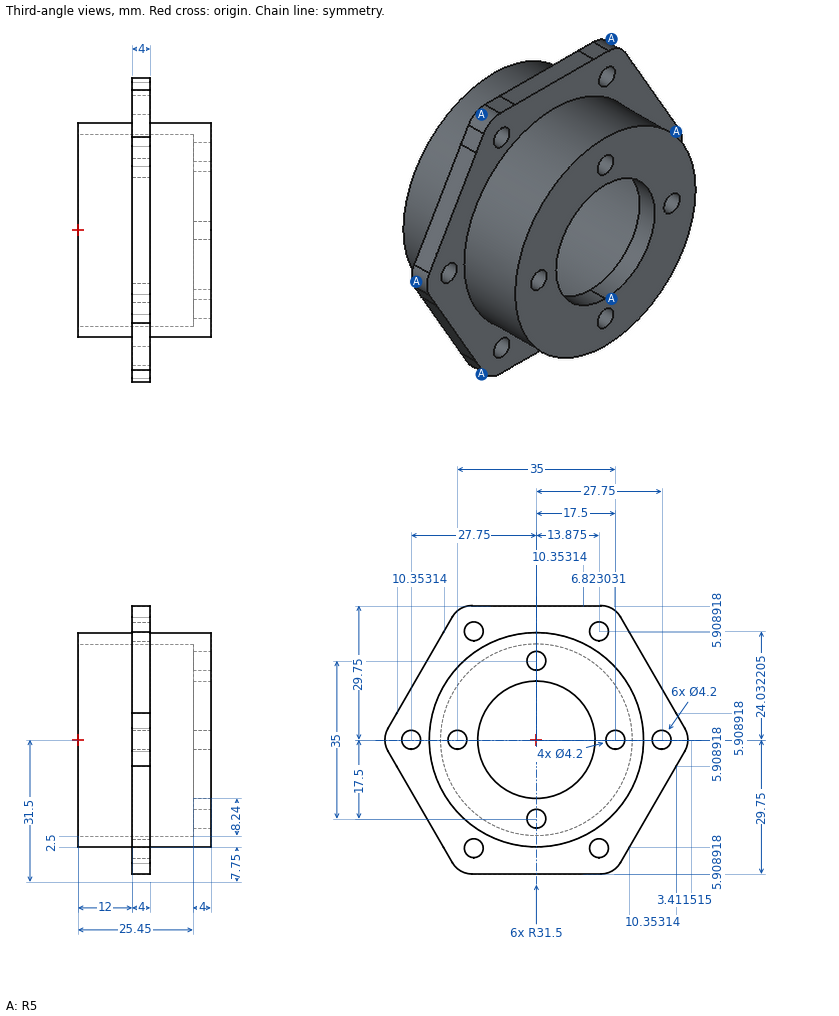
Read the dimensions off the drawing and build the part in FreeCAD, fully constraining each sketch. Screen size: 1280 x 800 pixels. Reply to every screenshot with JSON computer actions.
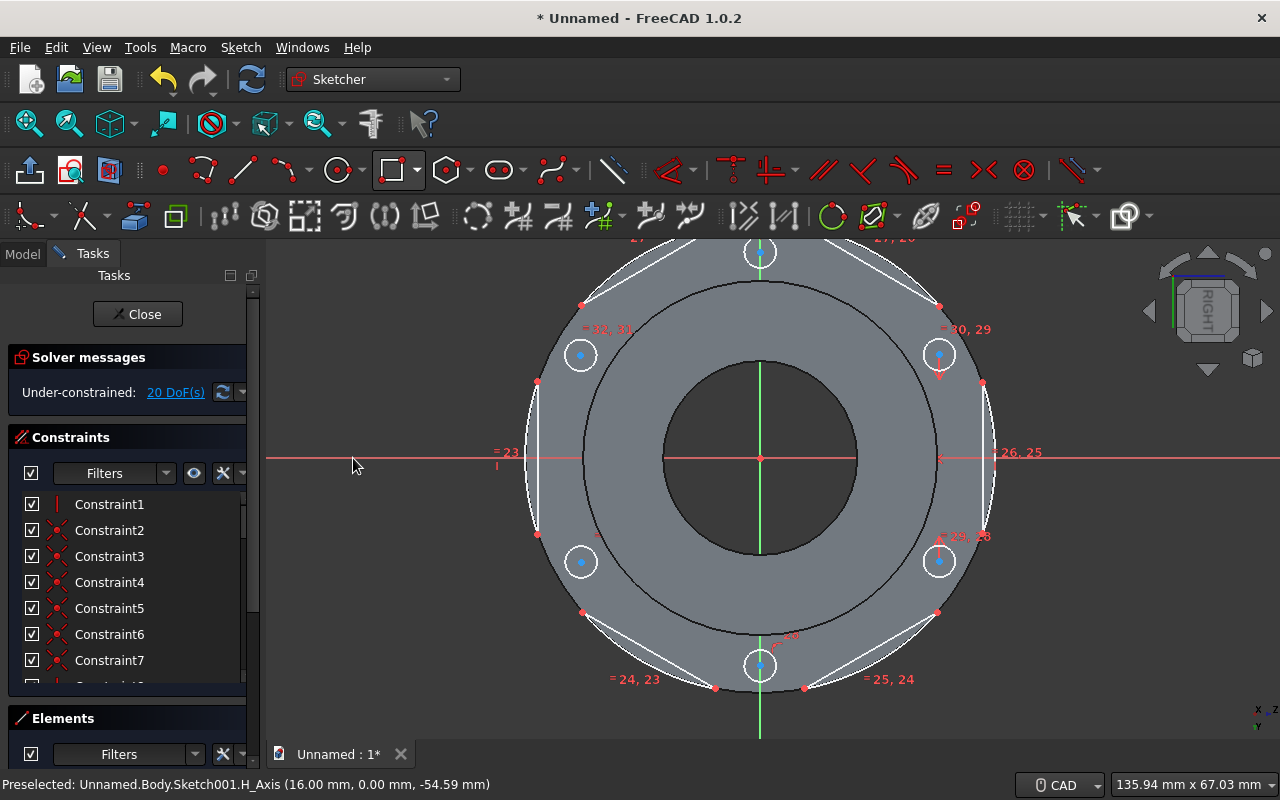
{"action": "left_click", "coordinate": [939, 355]}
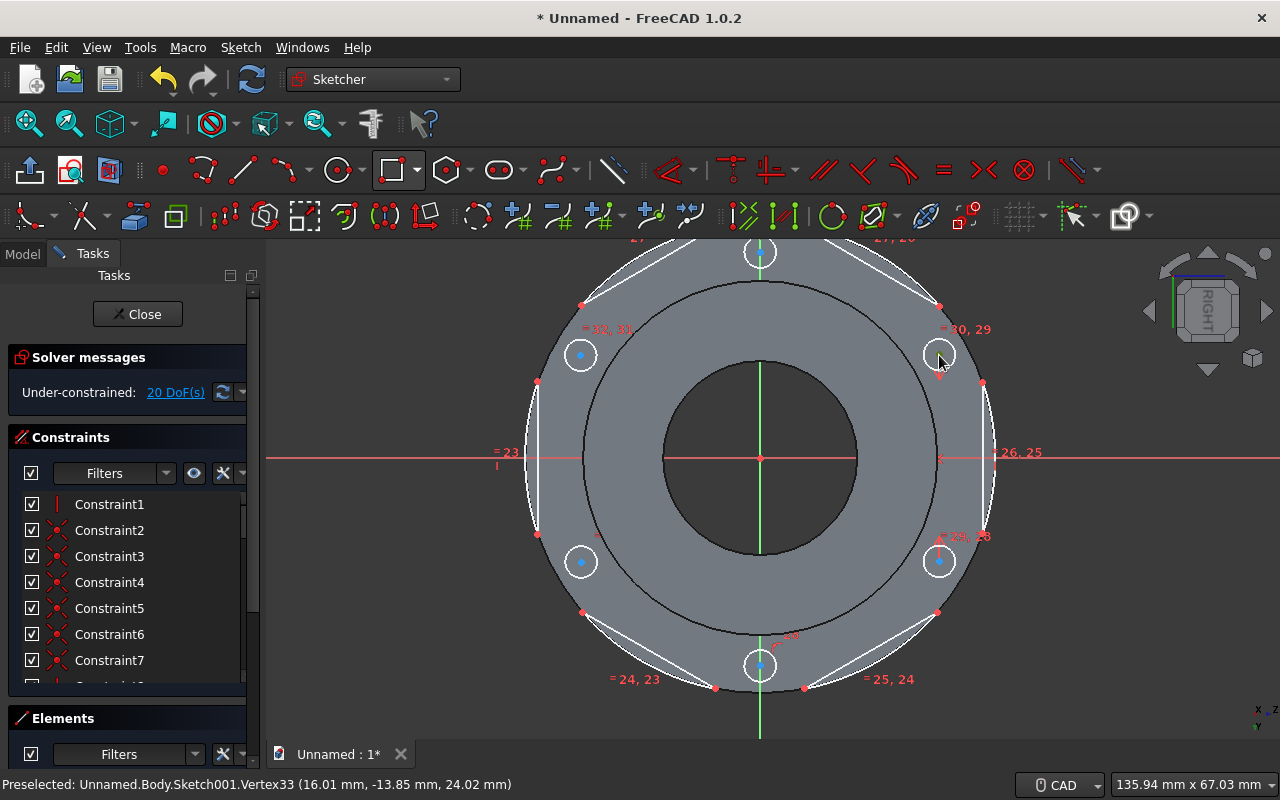
{"action": "left_click", "coordinate": [581, 355]}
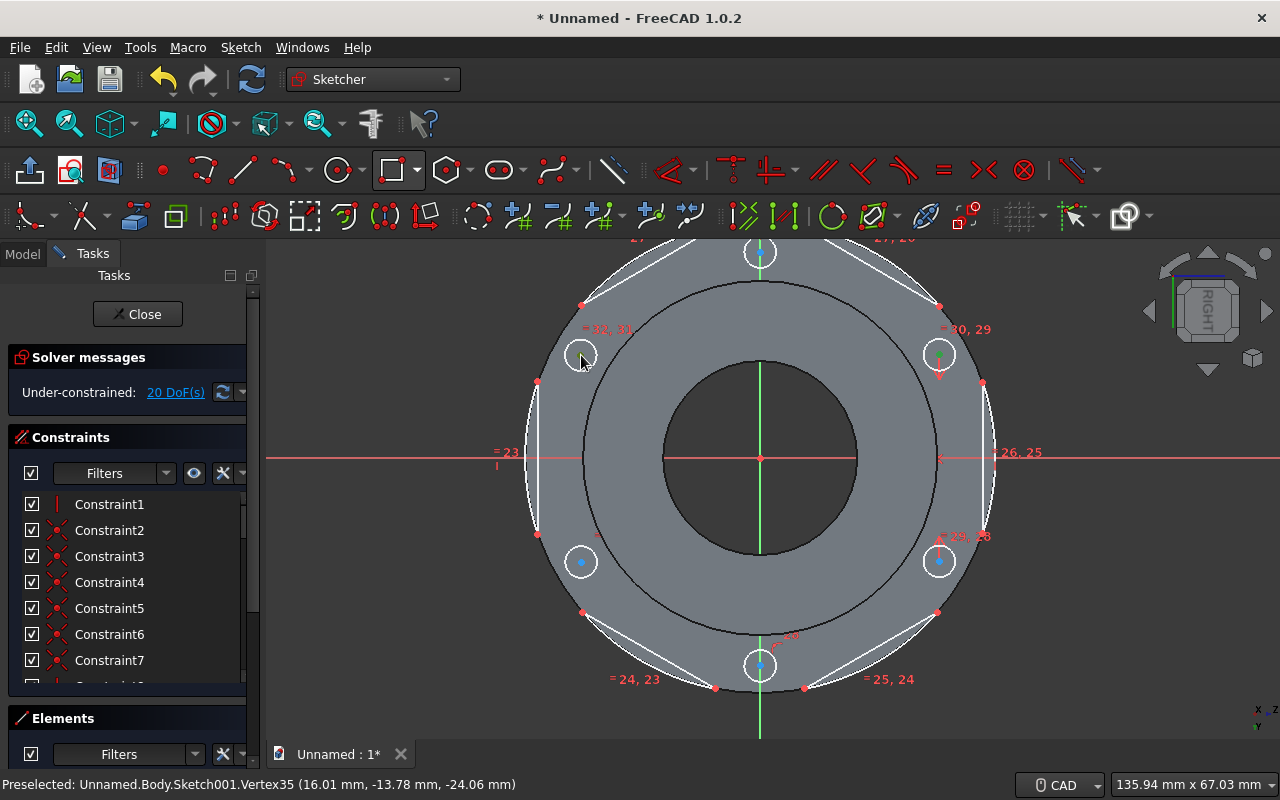
{"action": "left_click", "coordinate": [760, 616]}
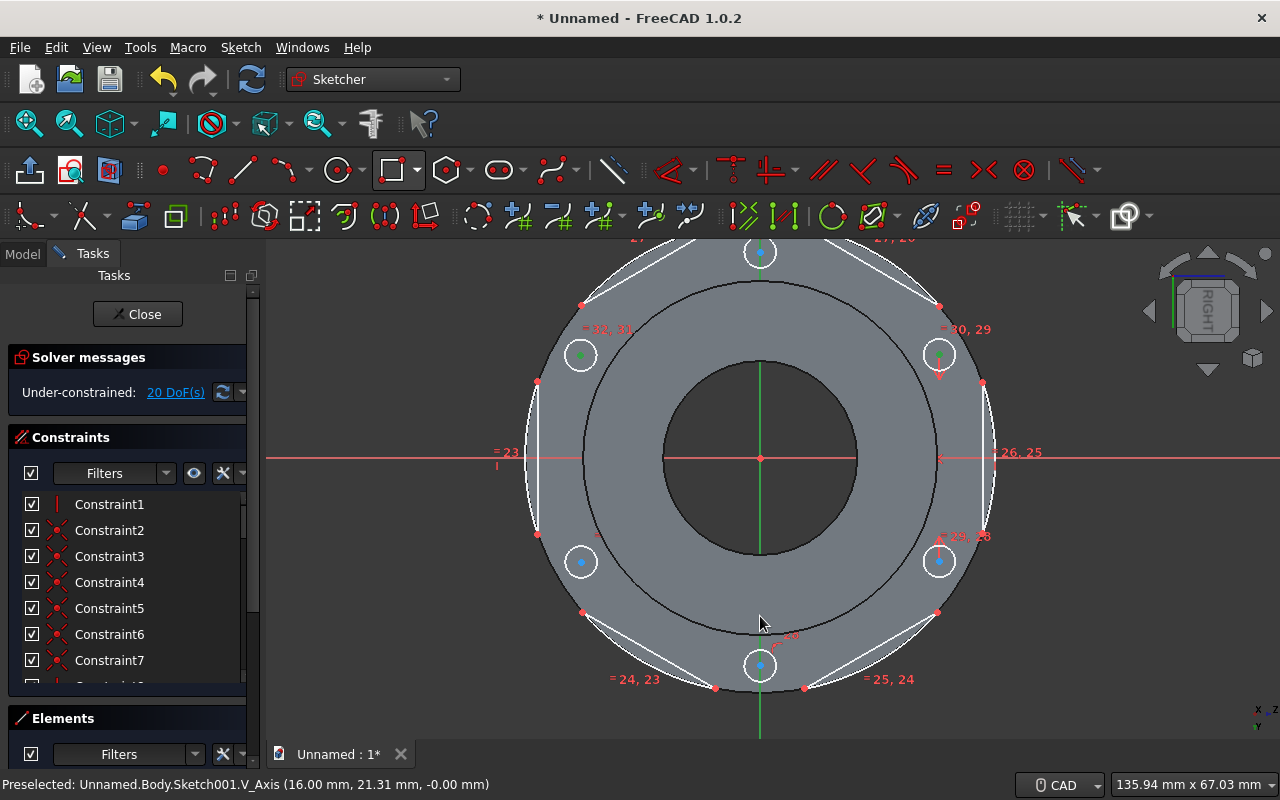
{"action": "key", "text": "s"}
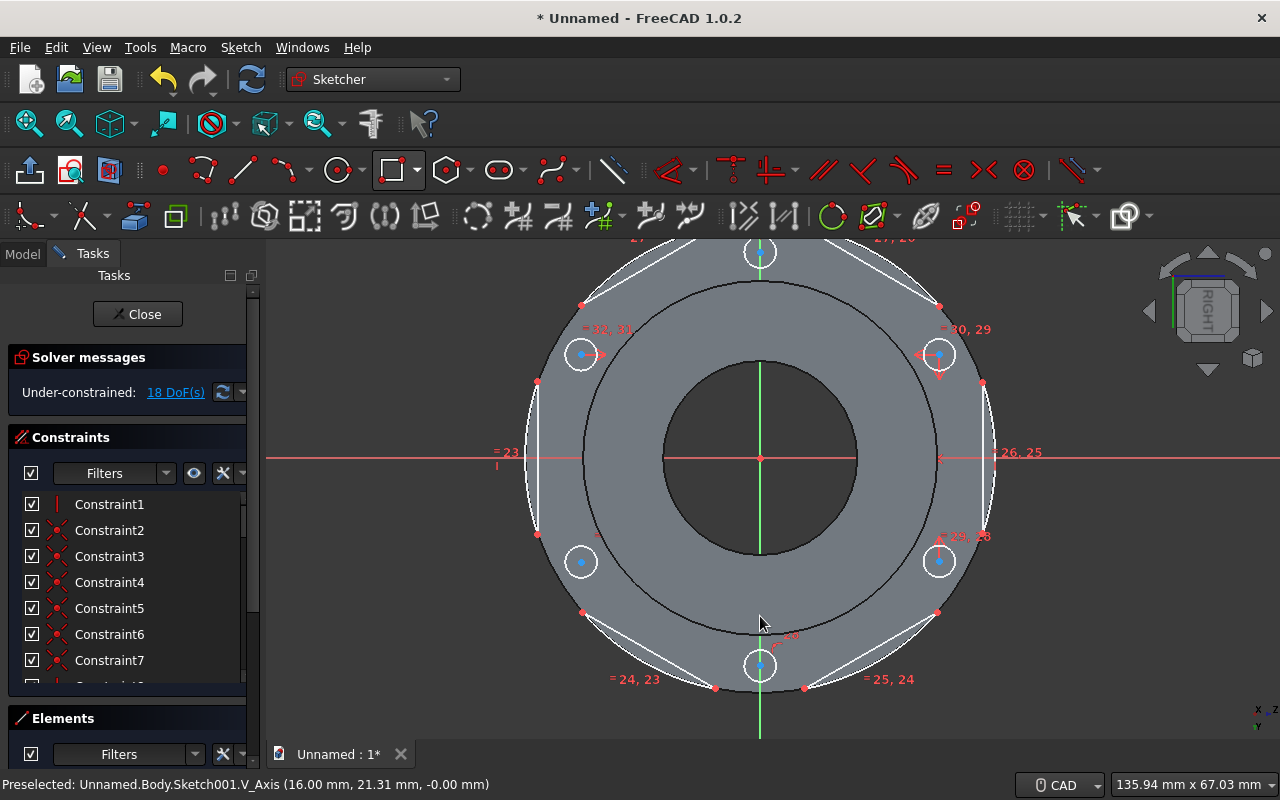
{"action": "left_click", "coordinate": [939, 561]}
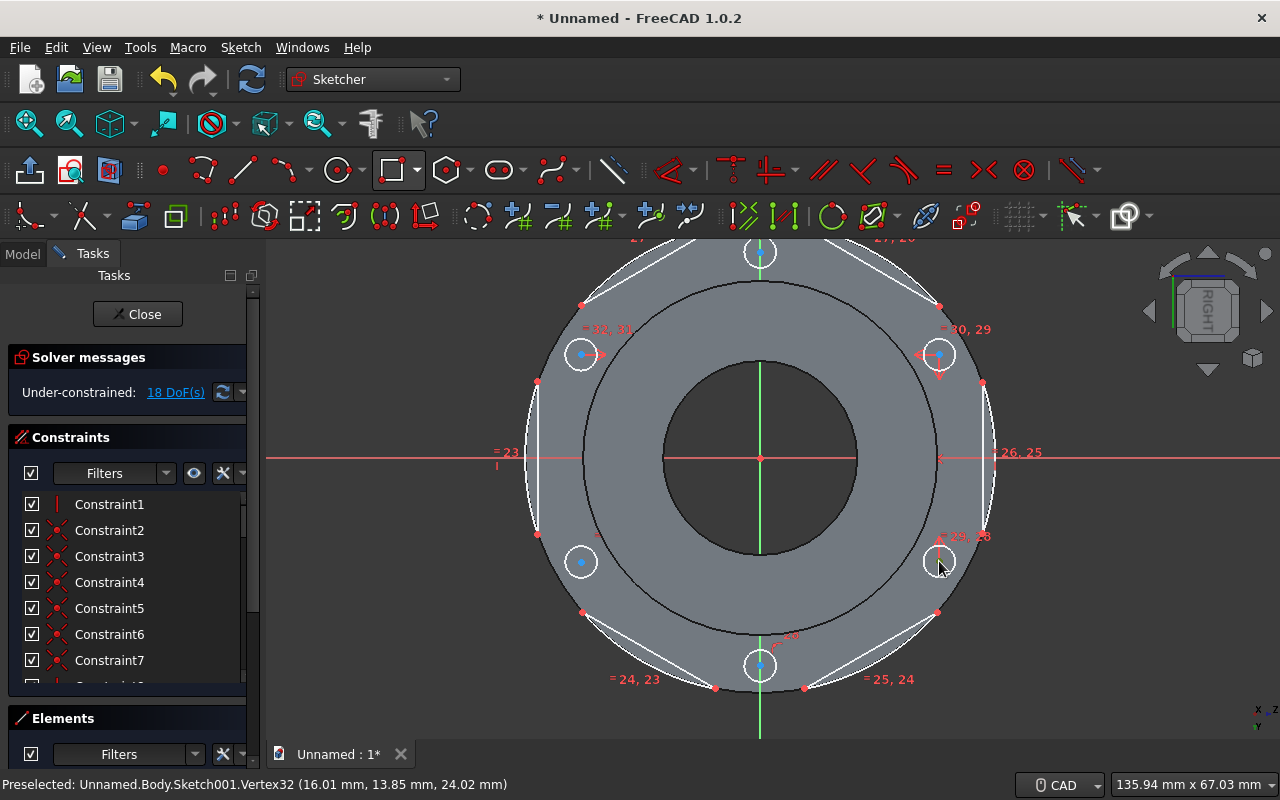
{"action": "left_click", "coordinate": [581, 562]}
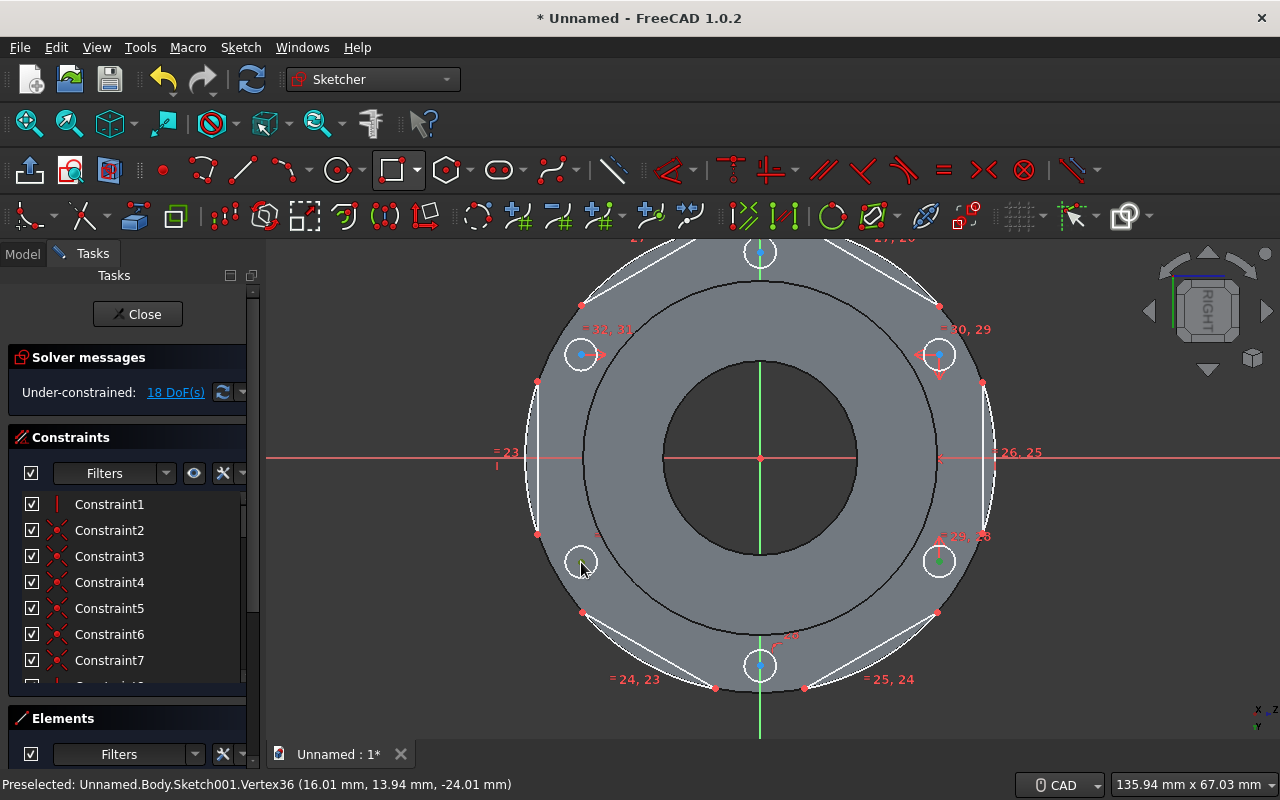
{"action": "left_click", "coordinate": [760, 616]}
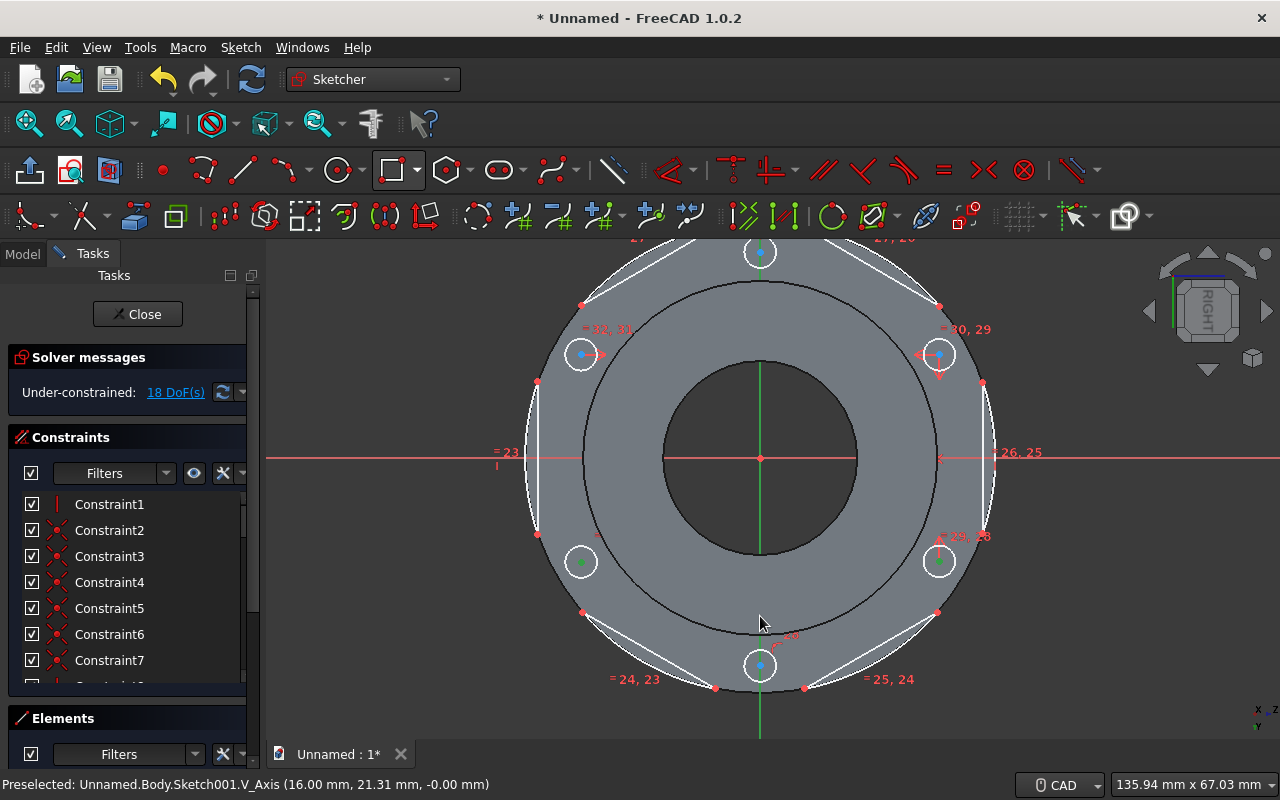
{"action": "left_click", "coordinate": [984, 170]}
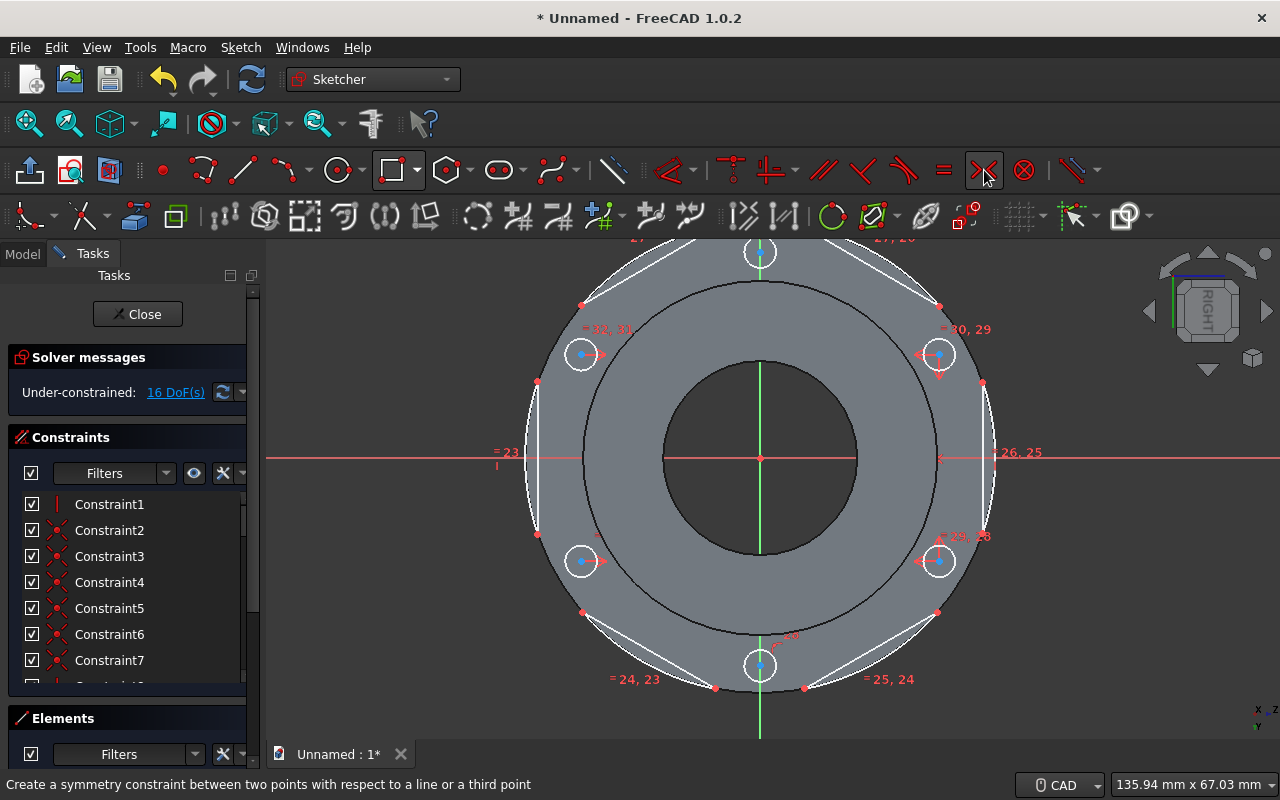
{"action": "left_click", "coordinate": [668, 170]}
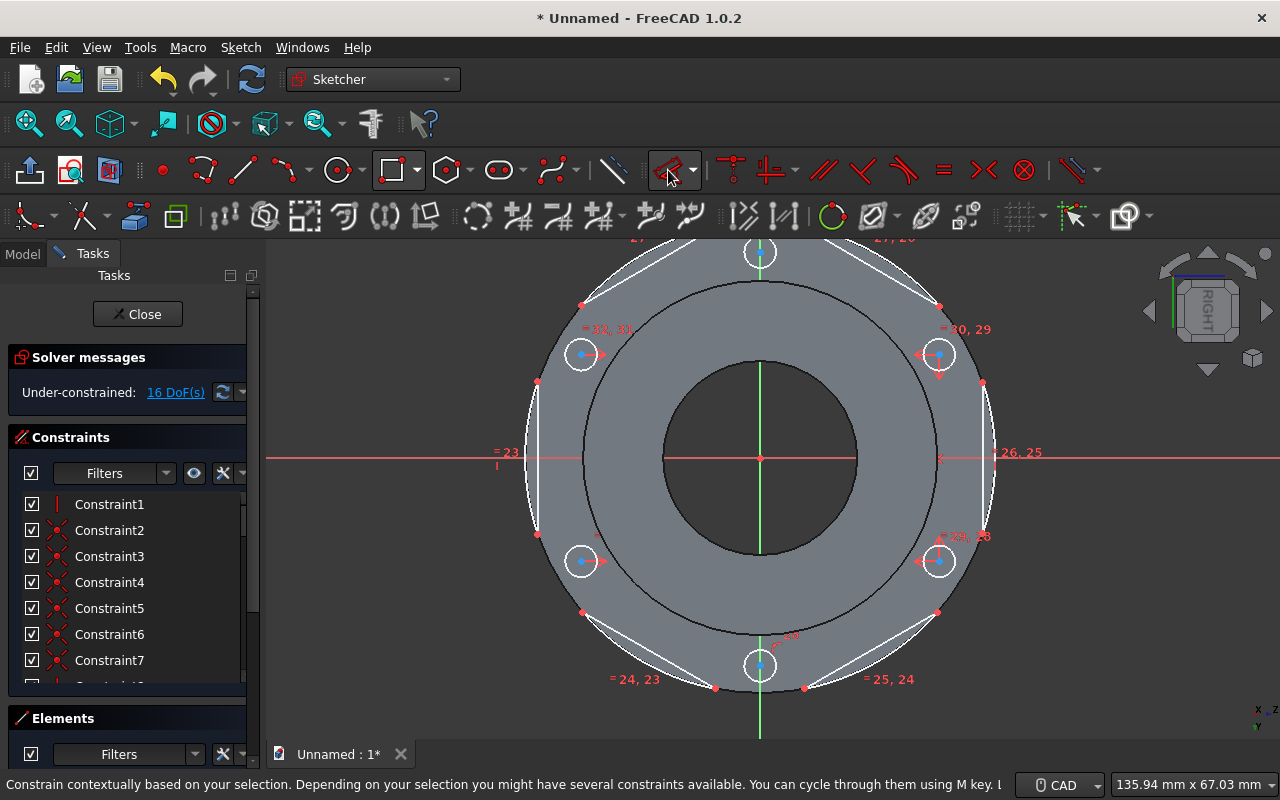
{"action": "scroll", "coordinate": [527, 427], "scroll_direction": "up", "scroll_amount": 2}